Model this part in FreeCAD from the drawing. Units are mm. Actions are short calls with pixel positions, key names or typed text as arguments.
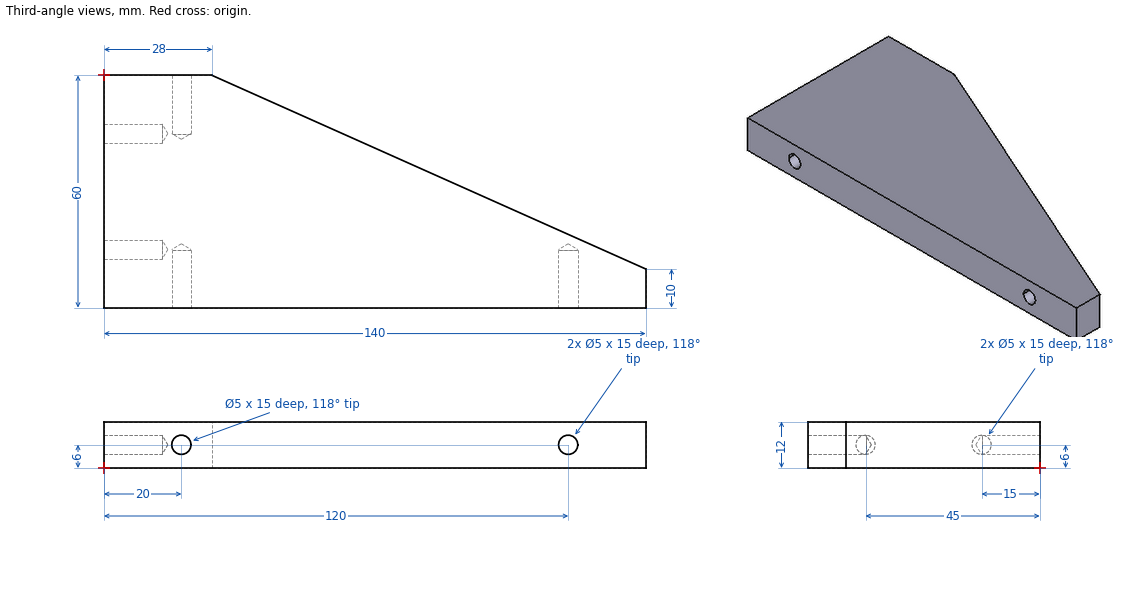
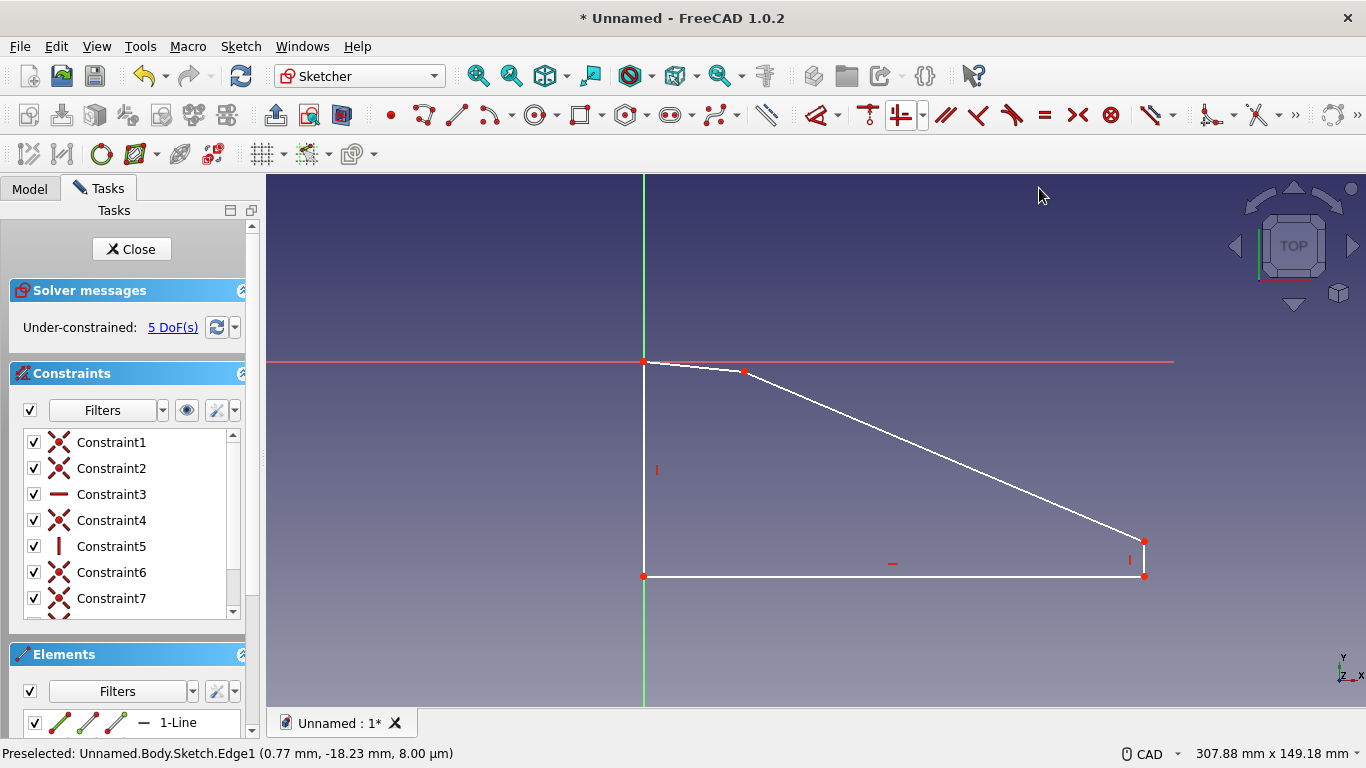
click(674, 365)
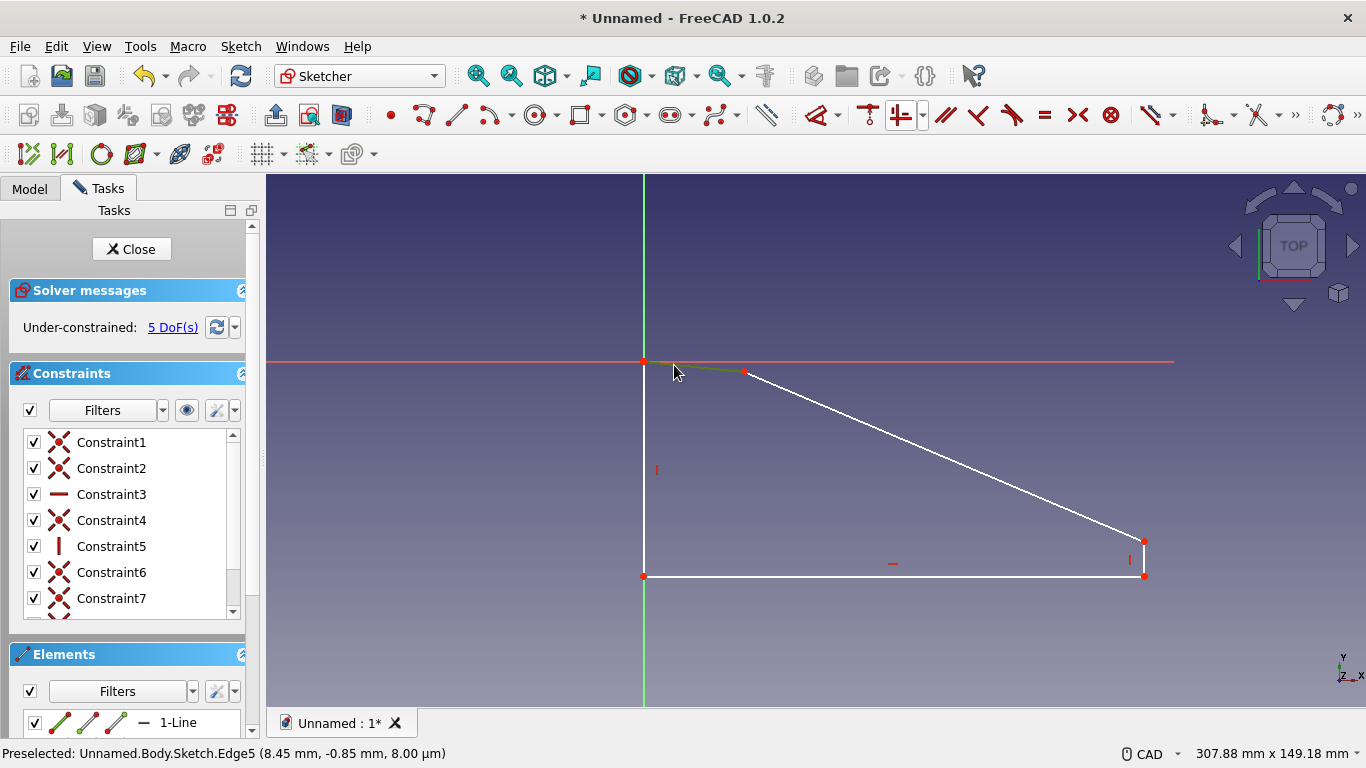
key(h)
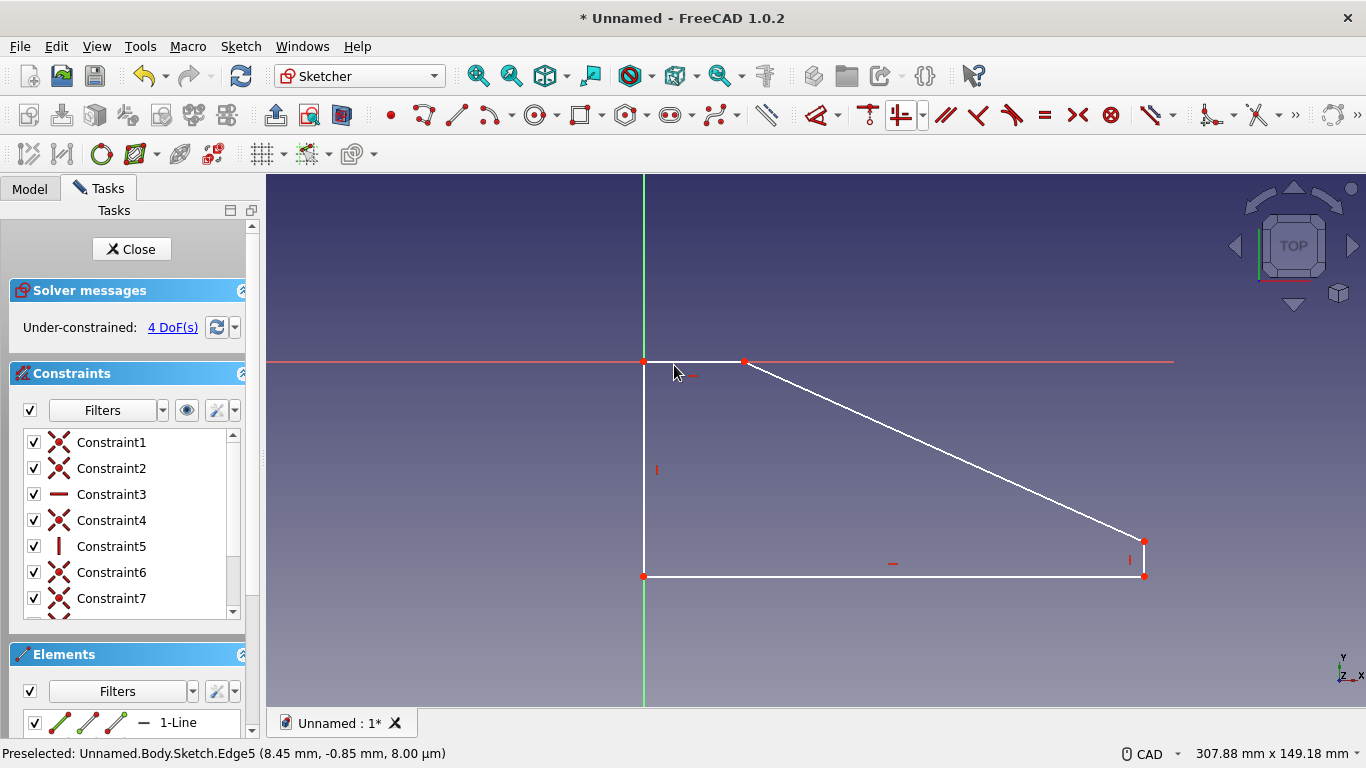
key(d)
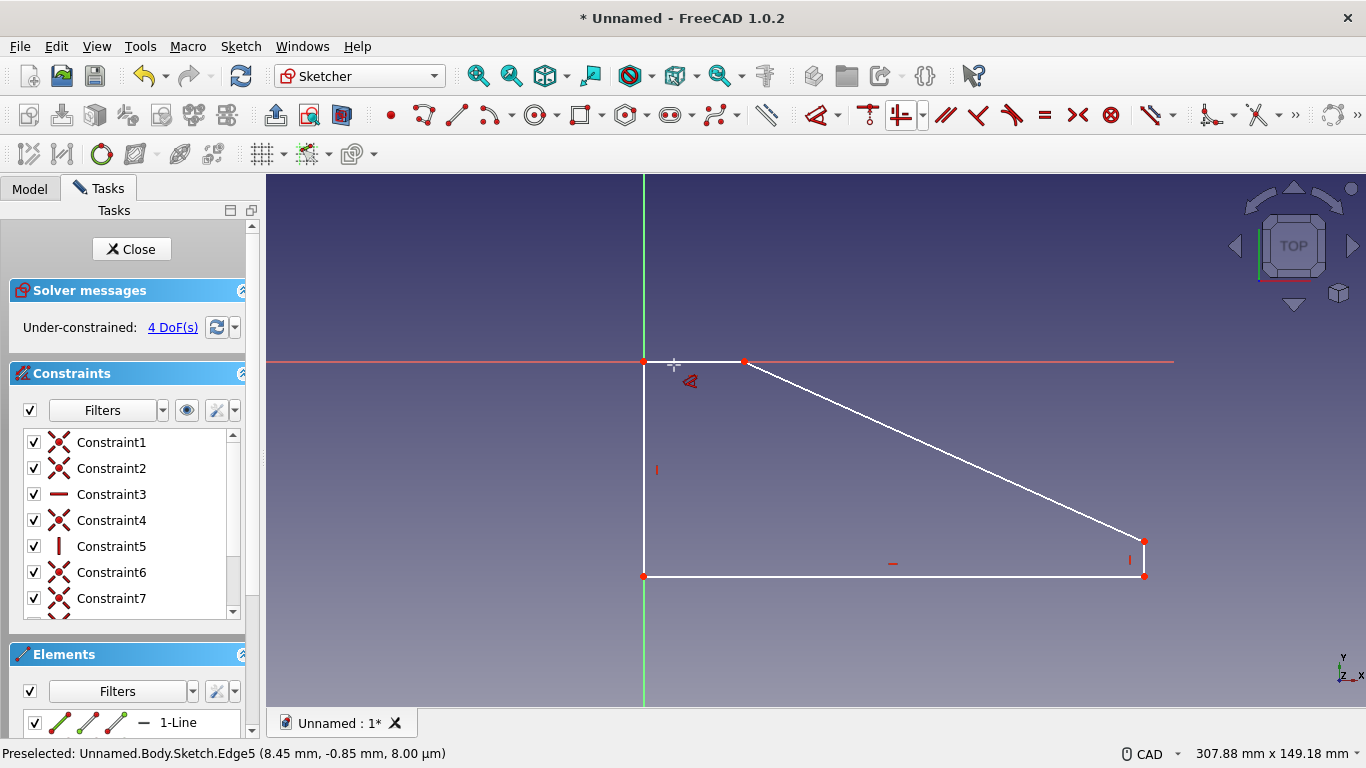
click(644, 426)
click(610, 469)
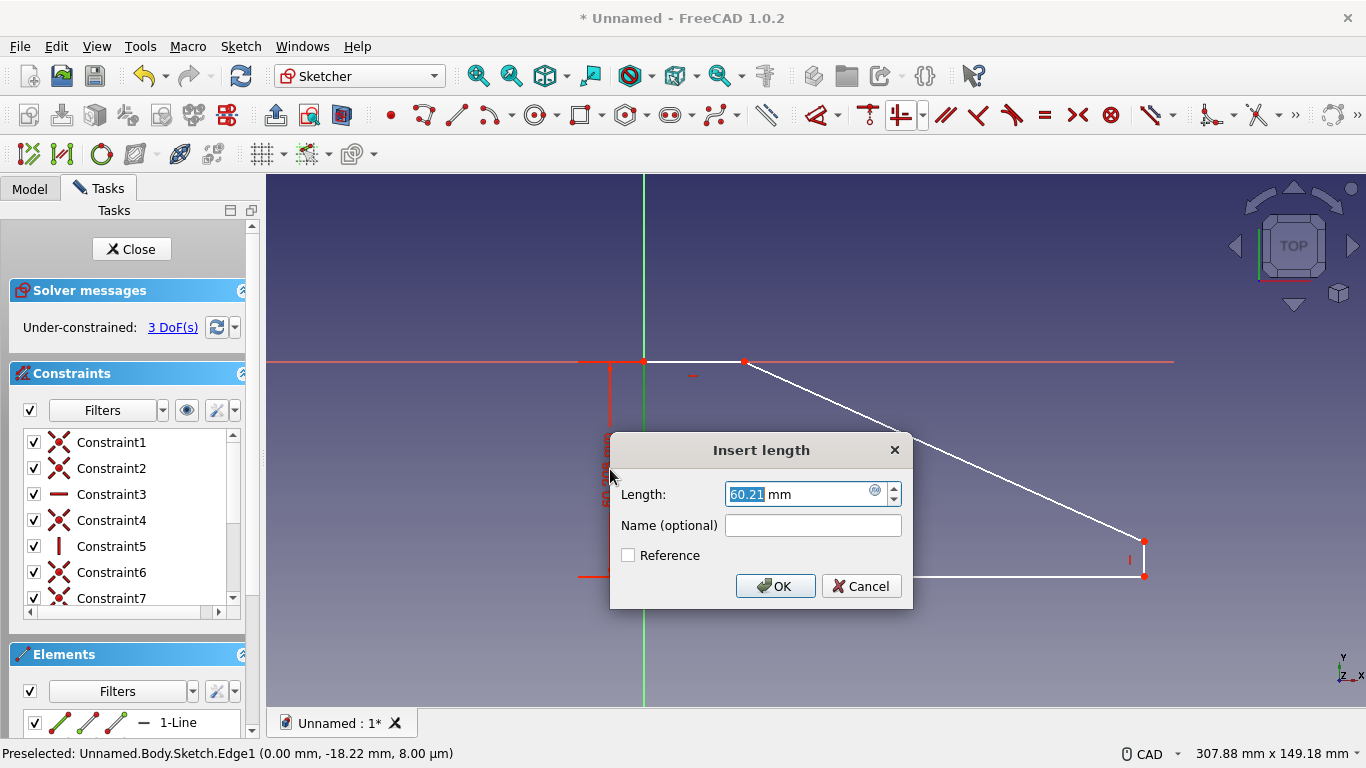
text(60)
key(Return)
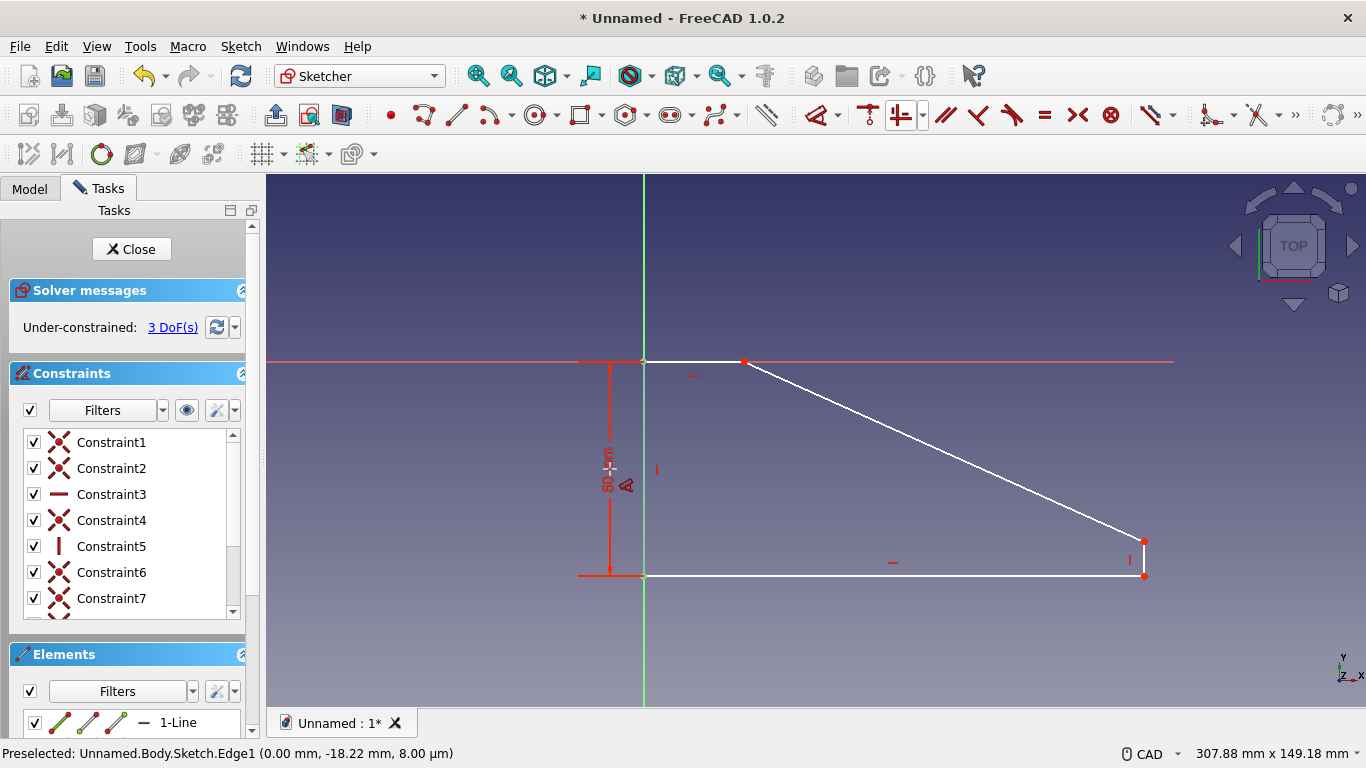
scroll(1144, 566, up, 2)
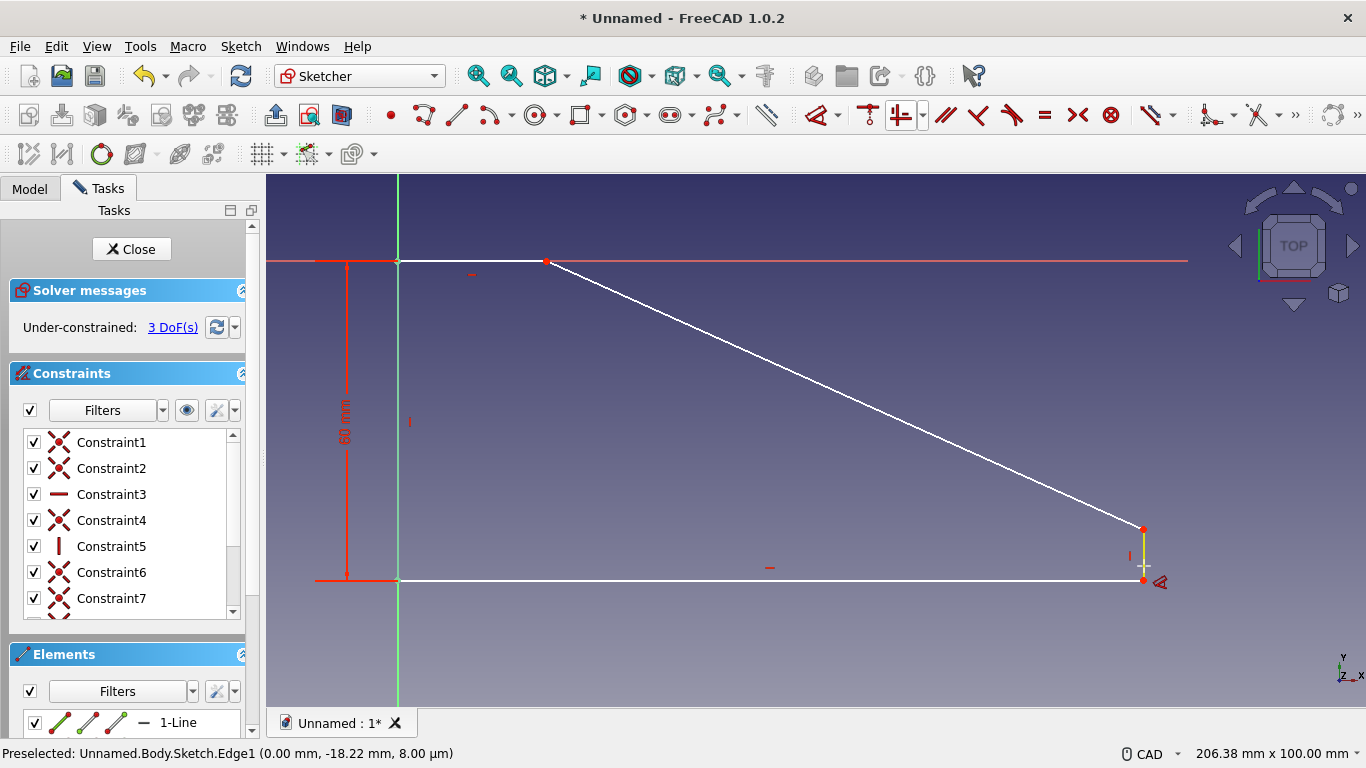
click(1144, 566)
click(1178, 555)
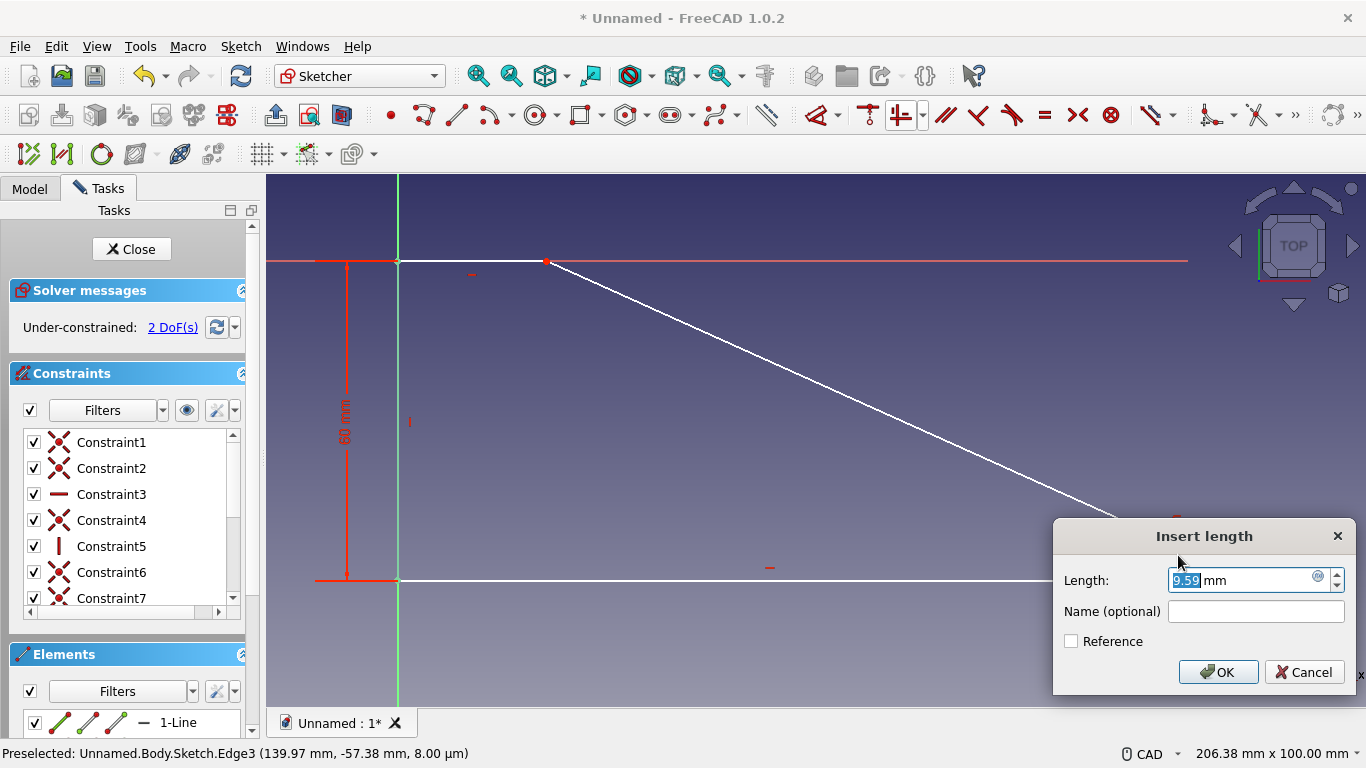
text(10)
key(Return)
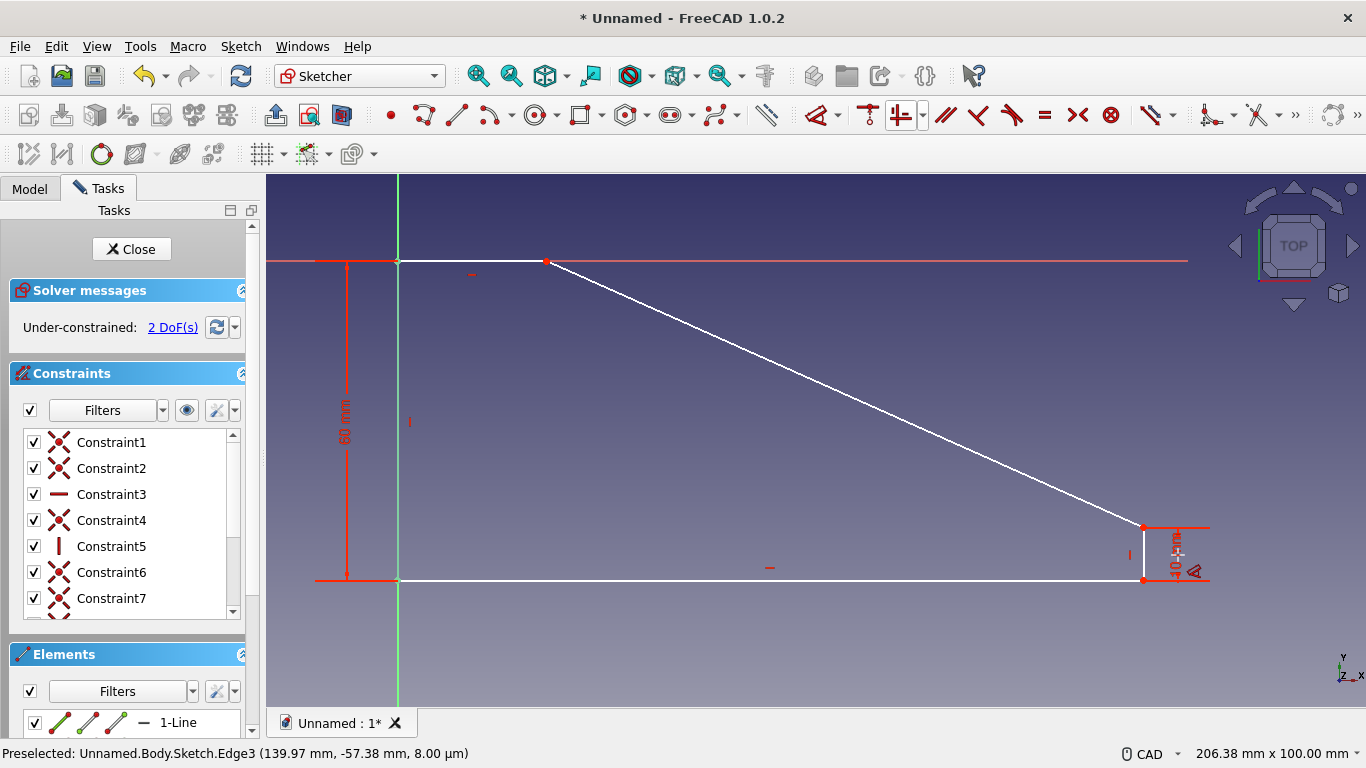
click(502, 261)
click(472, 227)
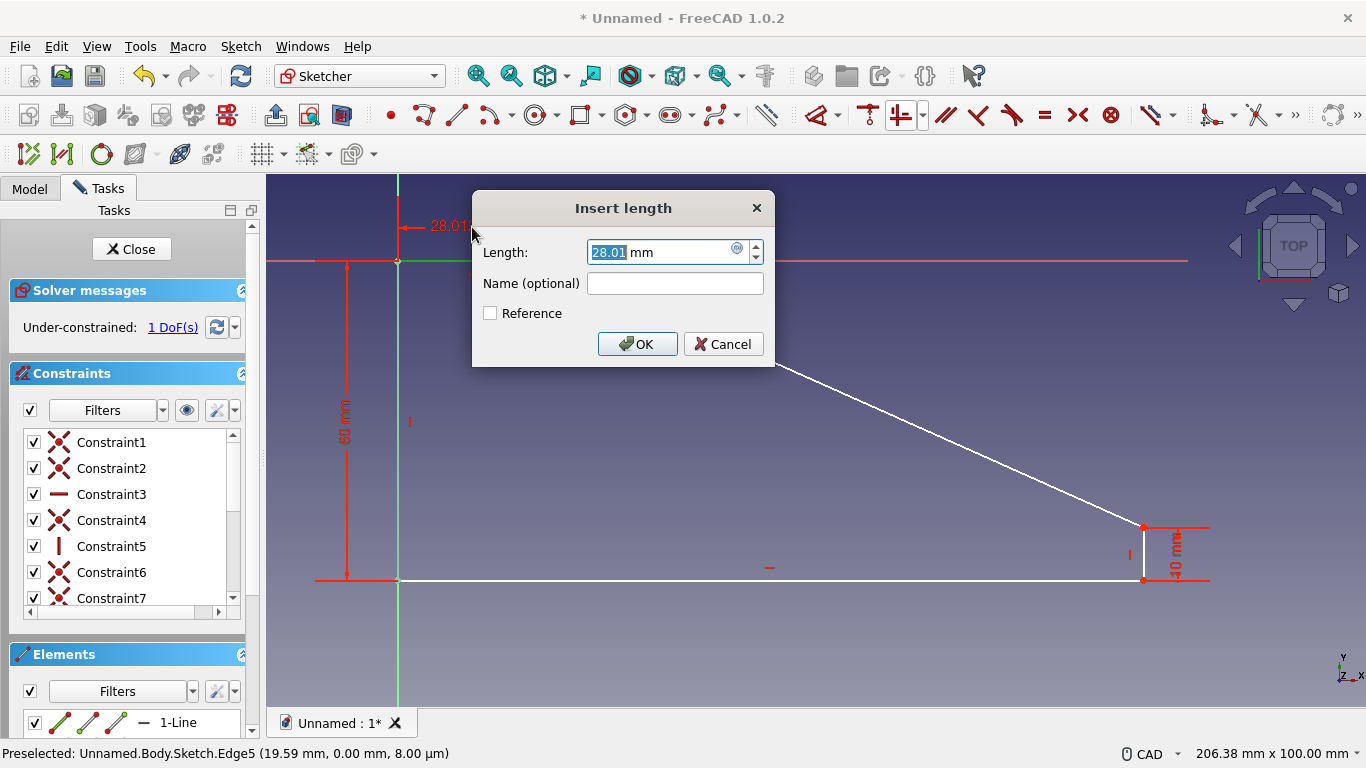
text(28)
key(Return)